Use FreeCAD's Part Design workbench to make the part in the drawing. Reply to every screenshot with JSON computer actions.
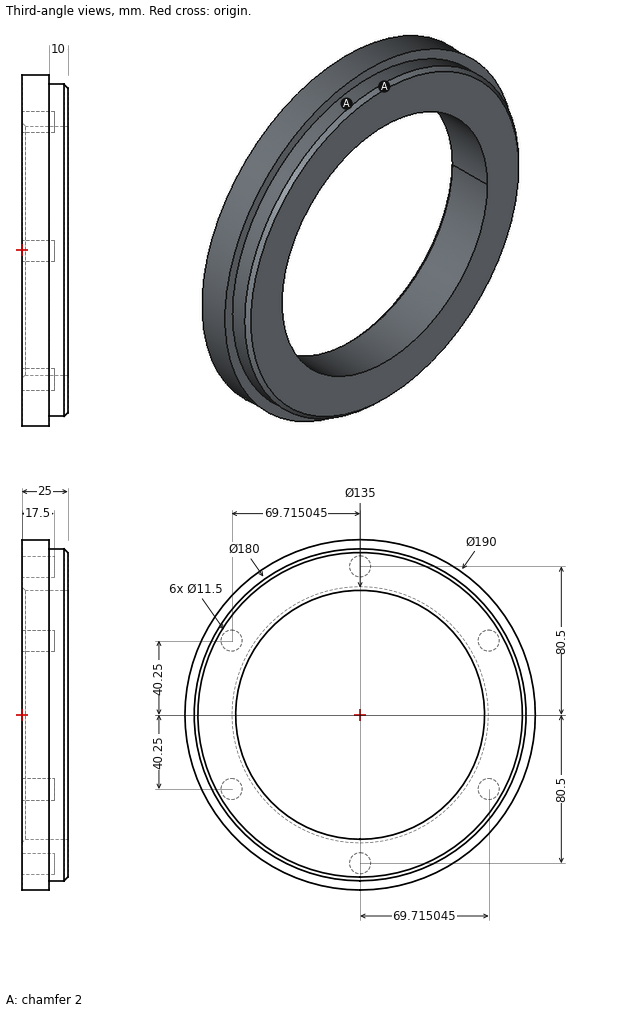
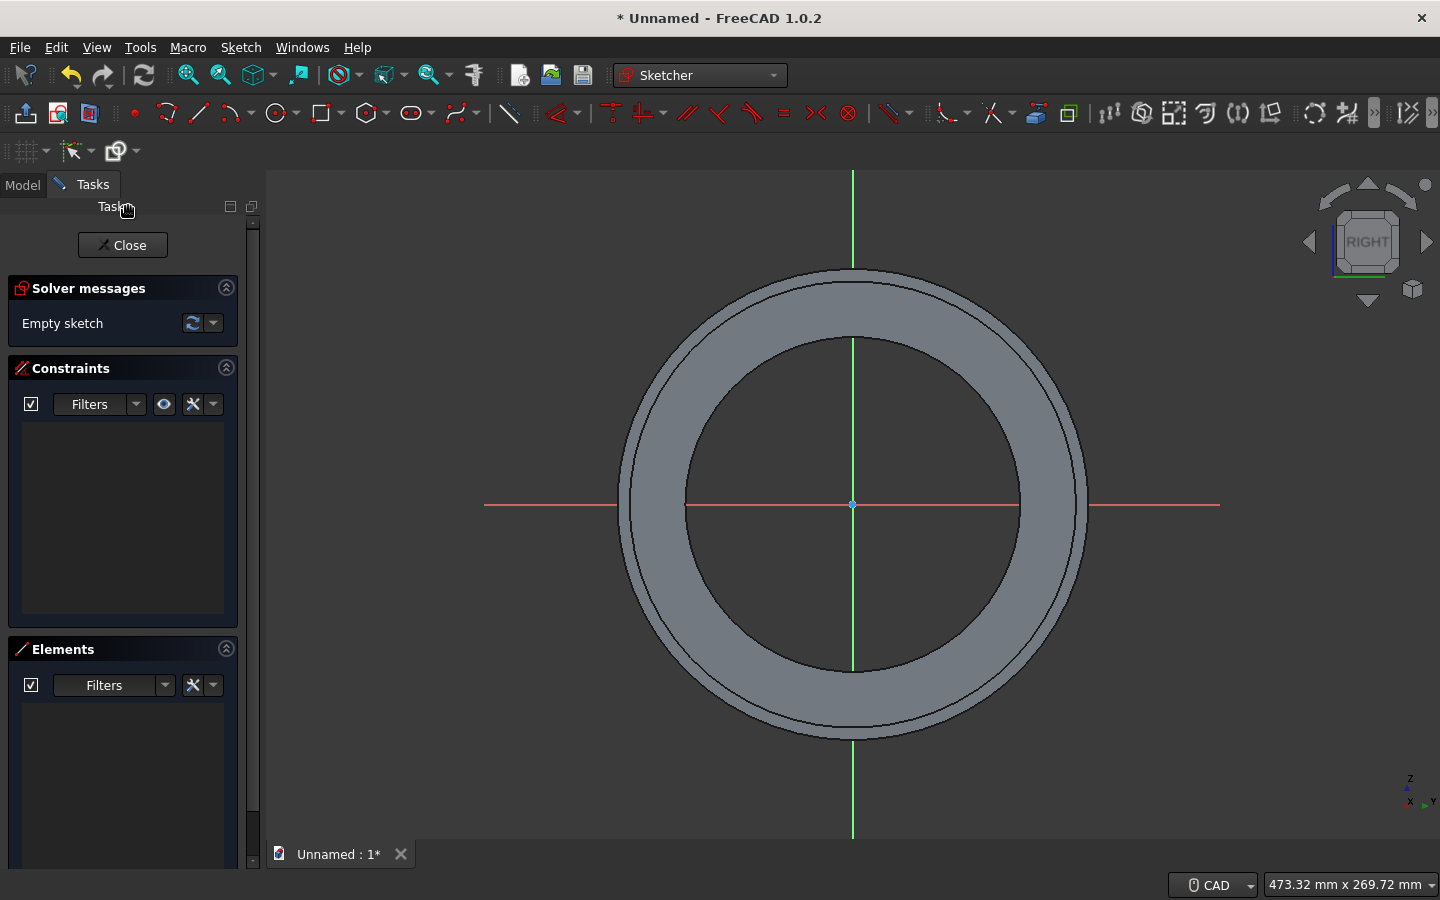
{"action": "left_click", "coordinate": [90, 114]}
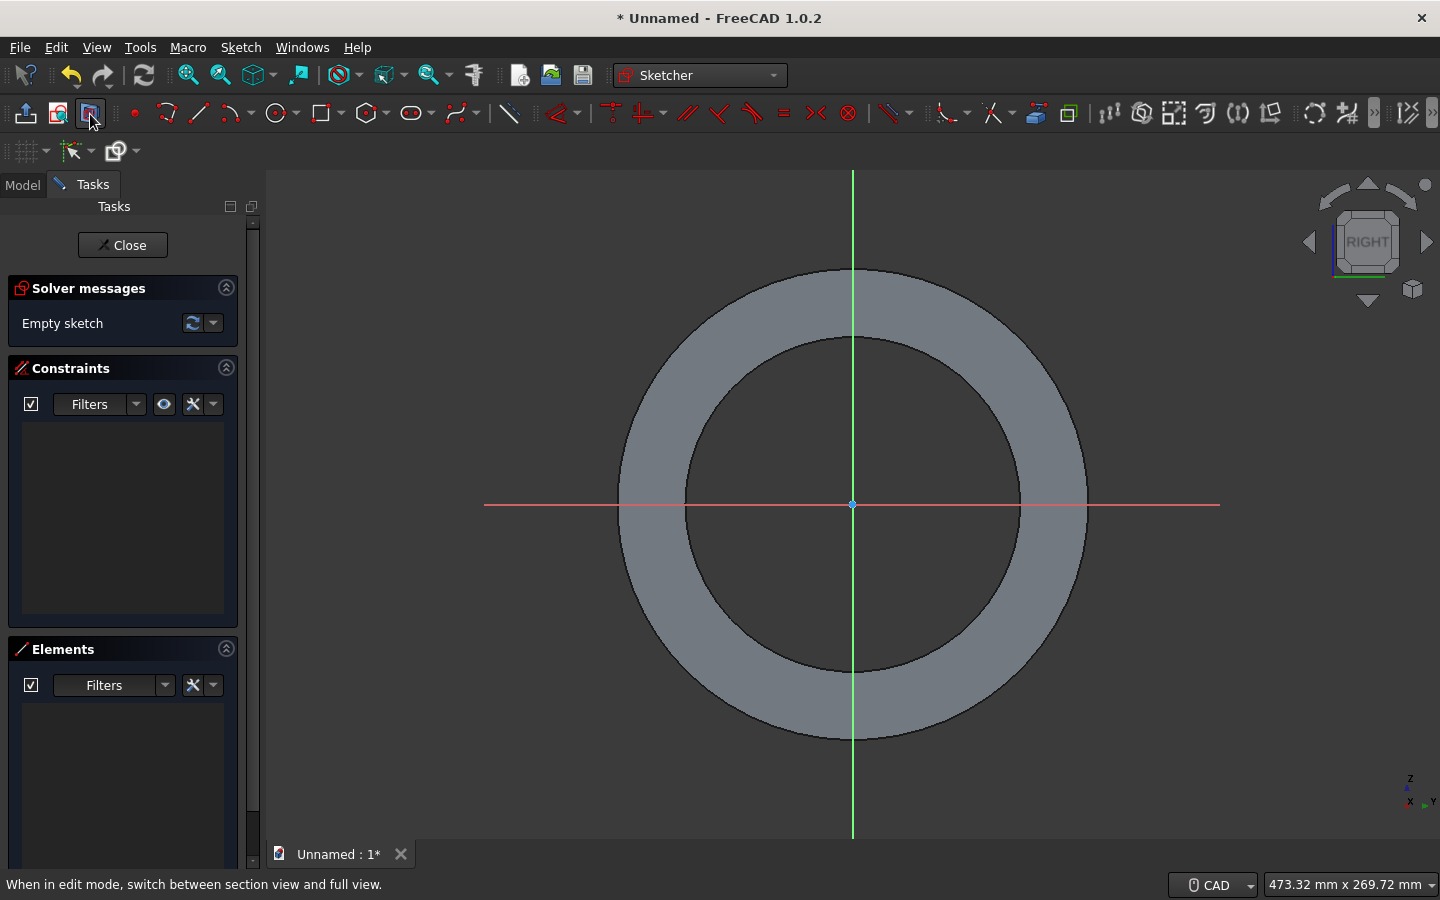
{"action": "left_click", "coordinate": [276, 114]}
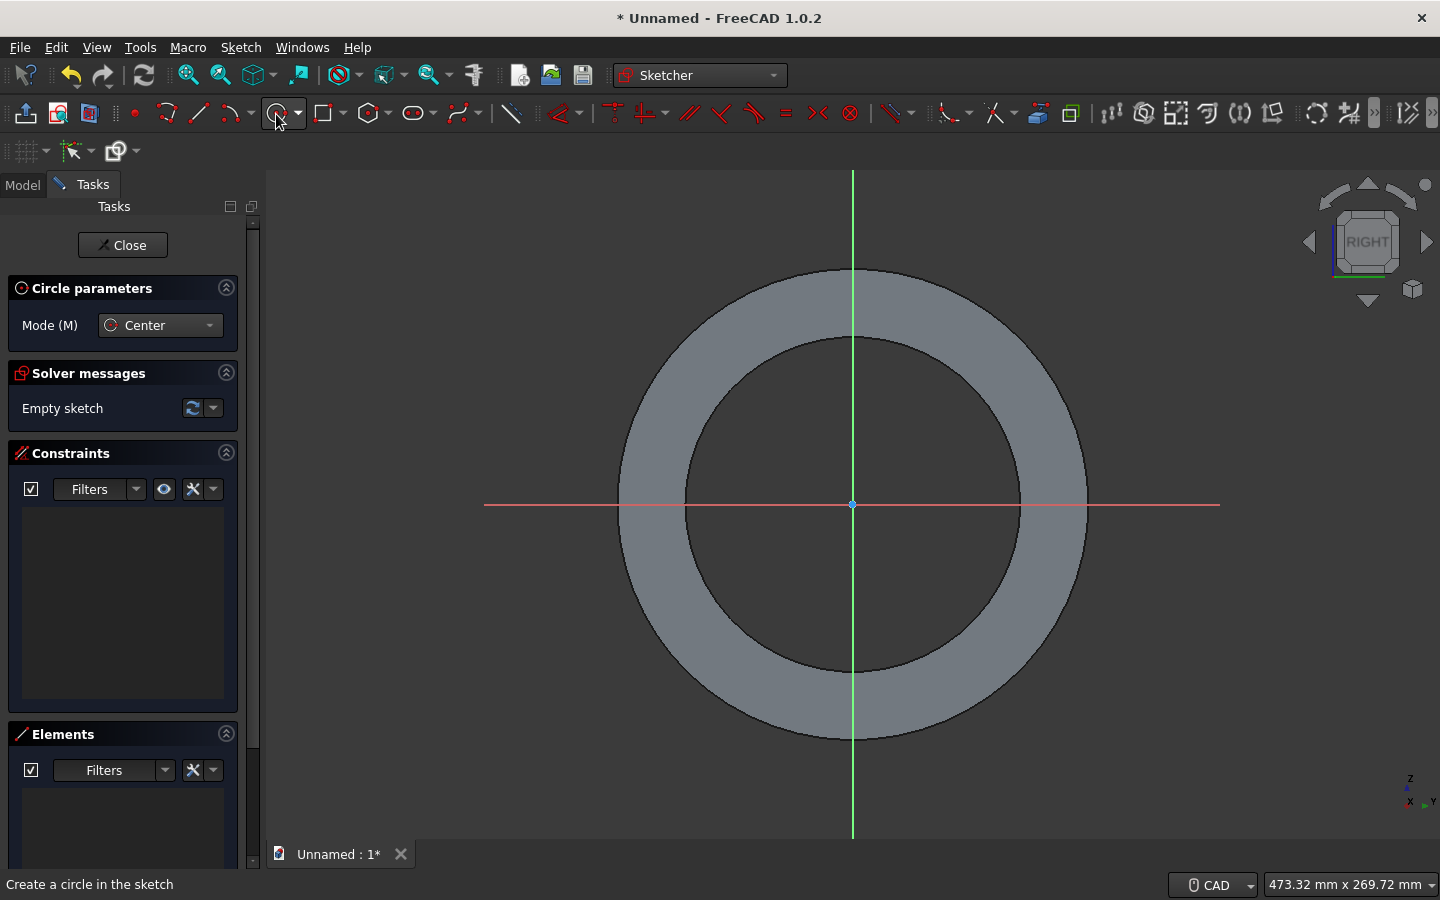
{"action": "scroll", "coordinate": [680, 405], "scroll_direction": "up", "scroll_amount": 3}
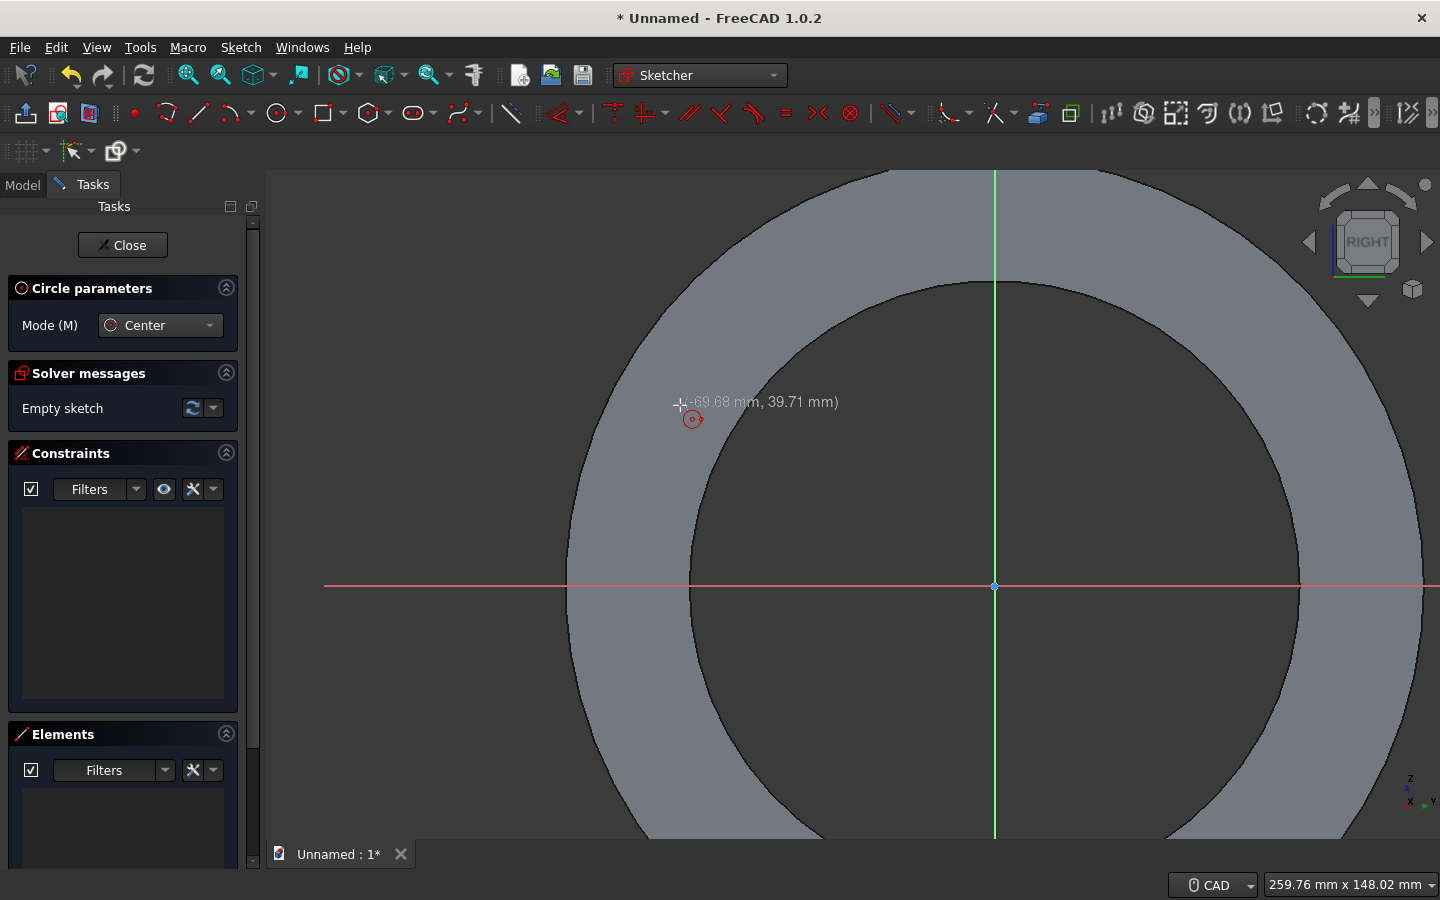
{"action": "left_click", "coordinate": [680, 404]}
{"action": "left_click", "coordinate": [698, 386]}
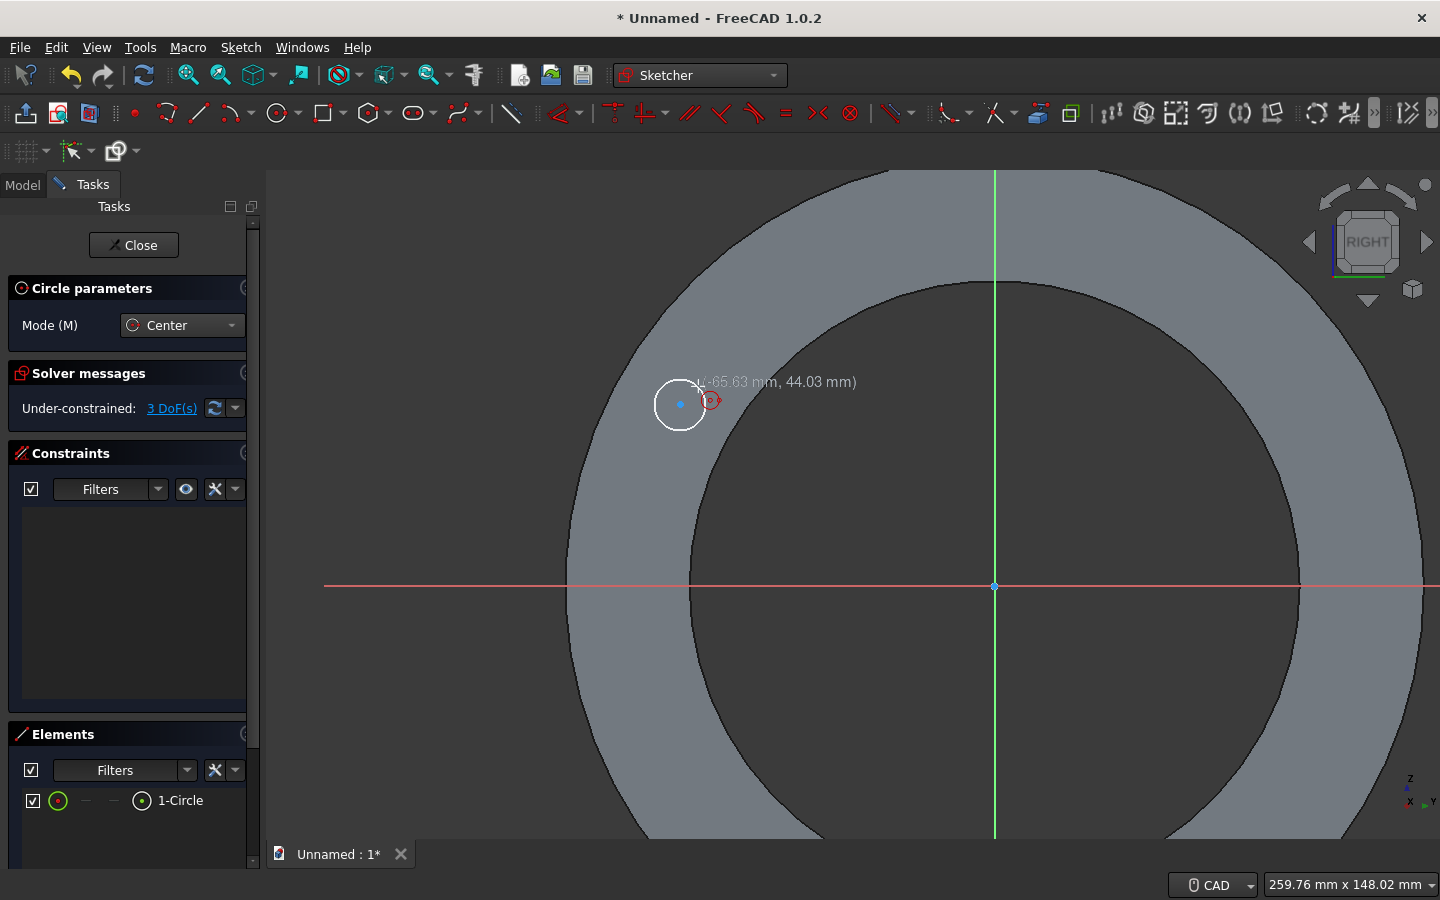
{"action": "left_click", "coordinate": [995, 222]}
{"action": "left_click", "coordinate": [1013, 204]}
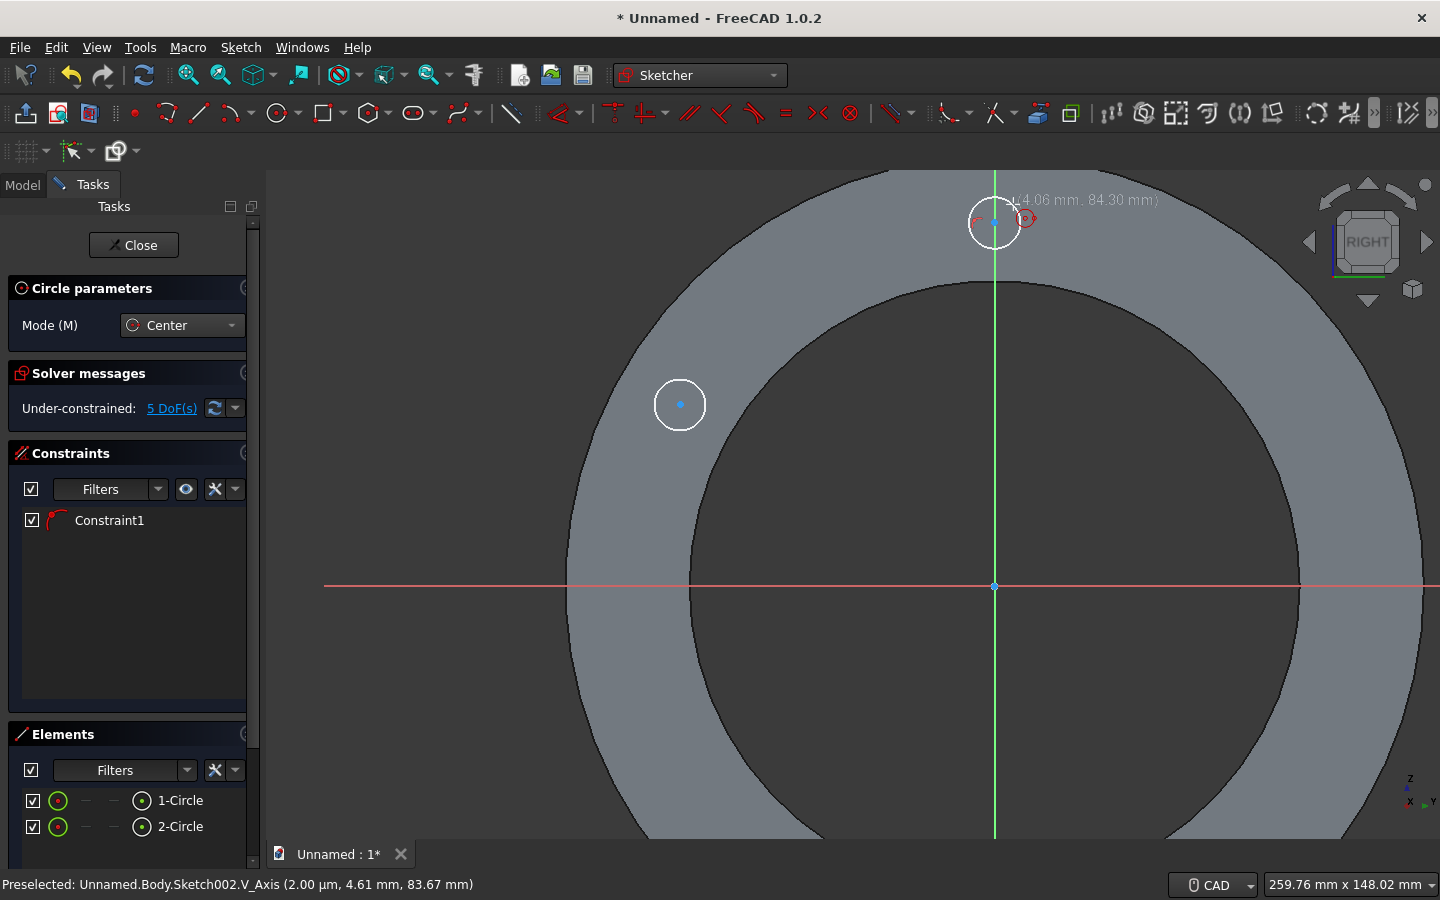
{"action": "left_click", "coordinate": [680, 768]}
{"action": "left_click", "coordinate": [698, 750]}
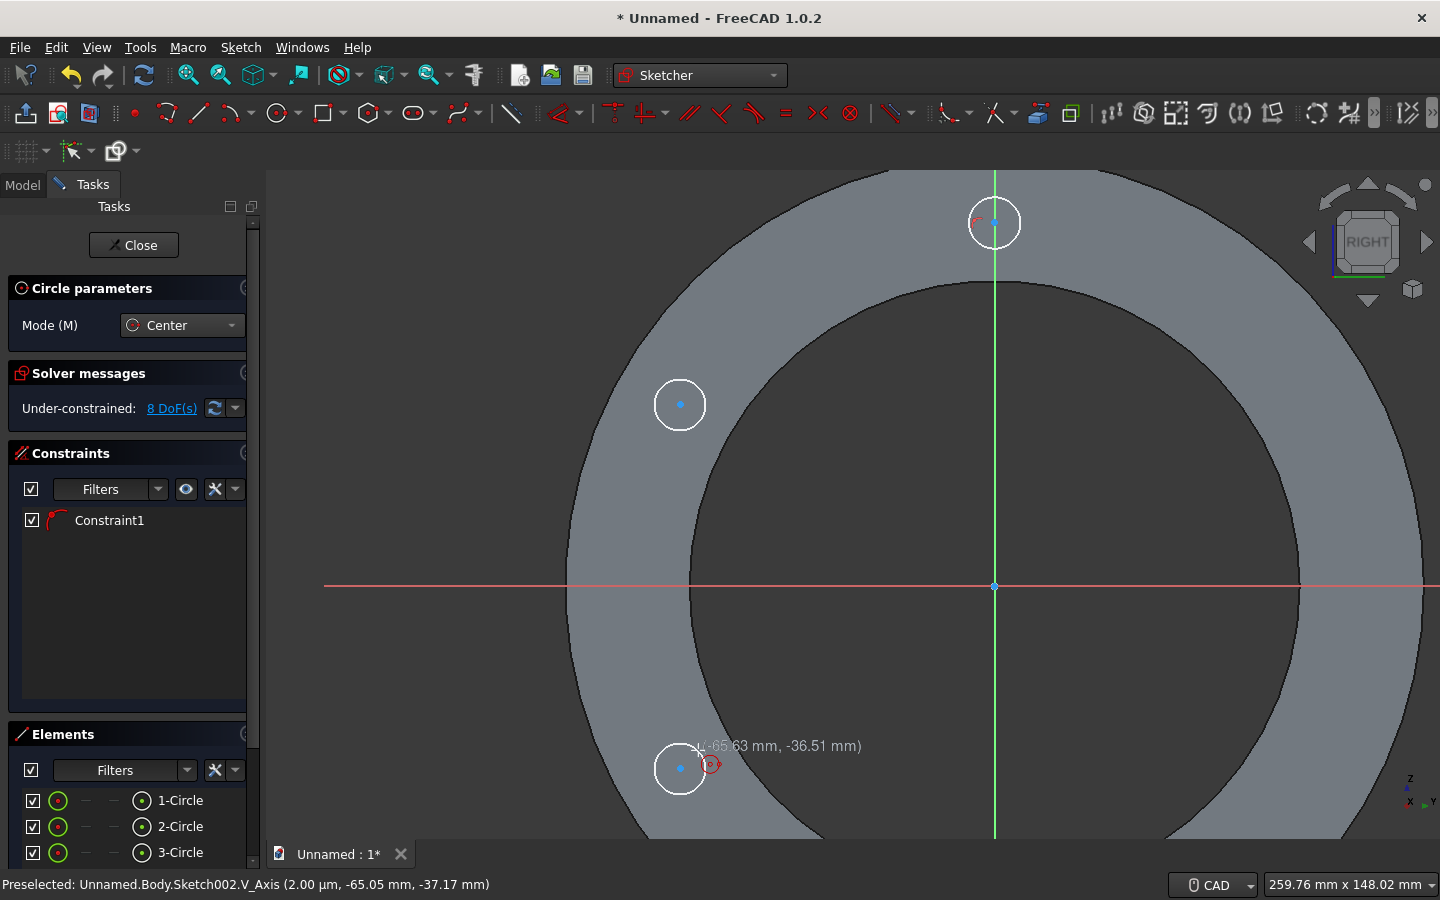
{"action": "scroll", "coordinate": [529, 405], "scroll_direction": "down", "scroll_amount": 3}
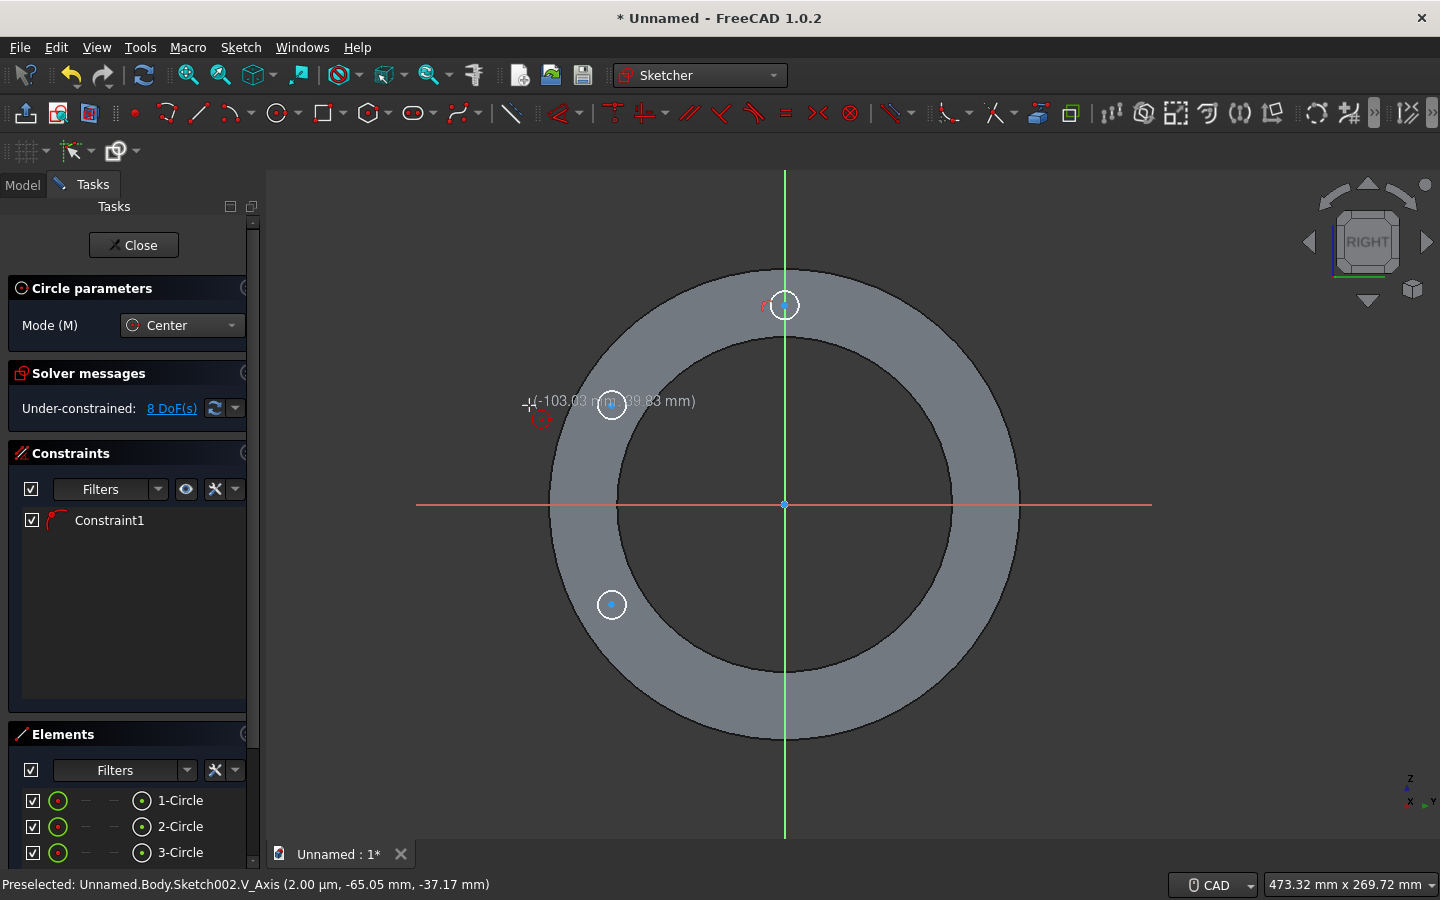
{"action": "scroll", "coordinate": [785, 704], "scroll_direction": "up", "scroll_amount": 3}